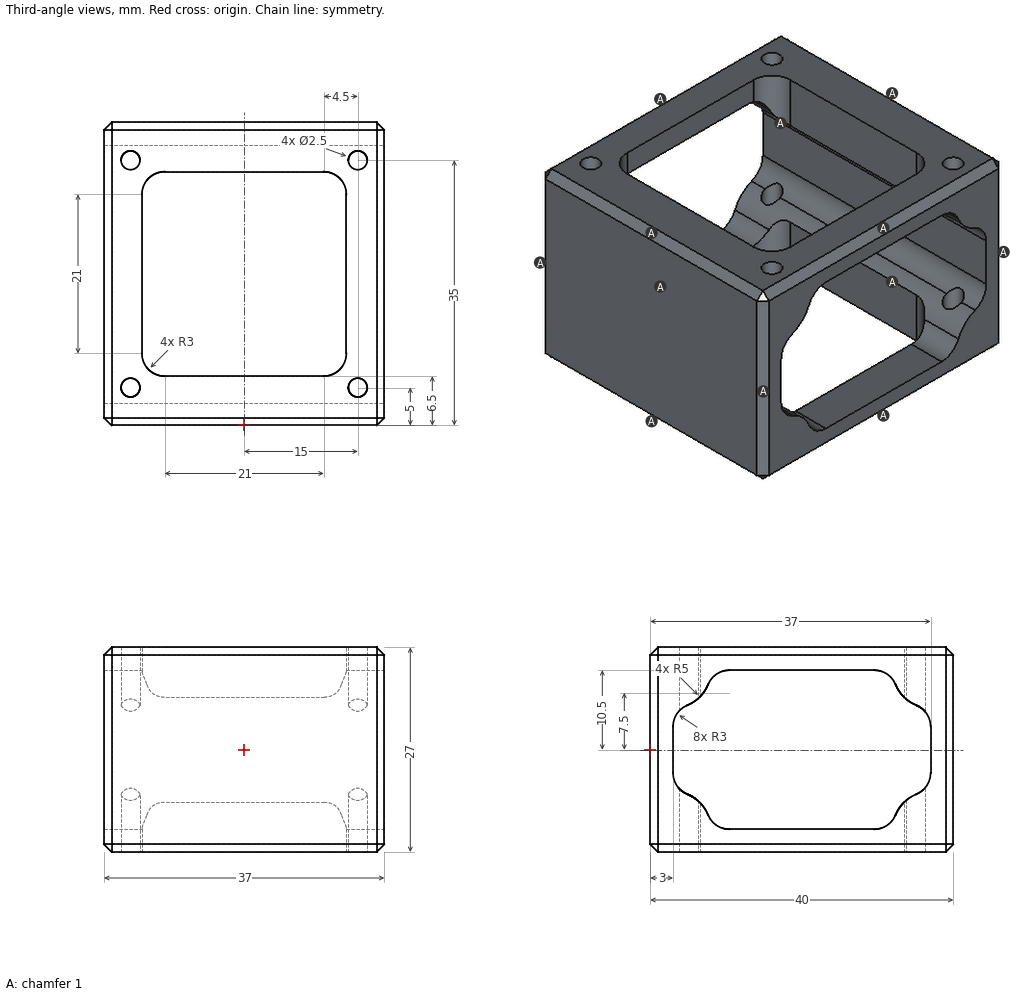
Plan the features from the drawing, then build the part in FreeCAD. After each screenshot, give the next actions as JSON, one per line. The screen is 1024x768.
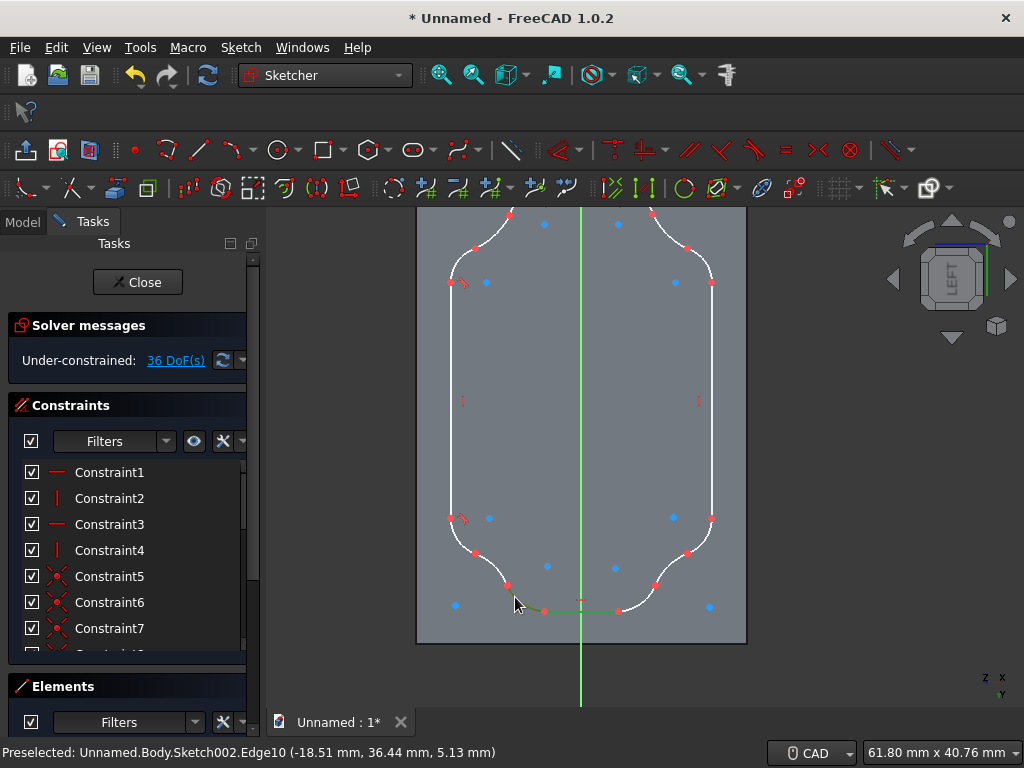
{"action": "left_click", "coordinate": [754, 150]}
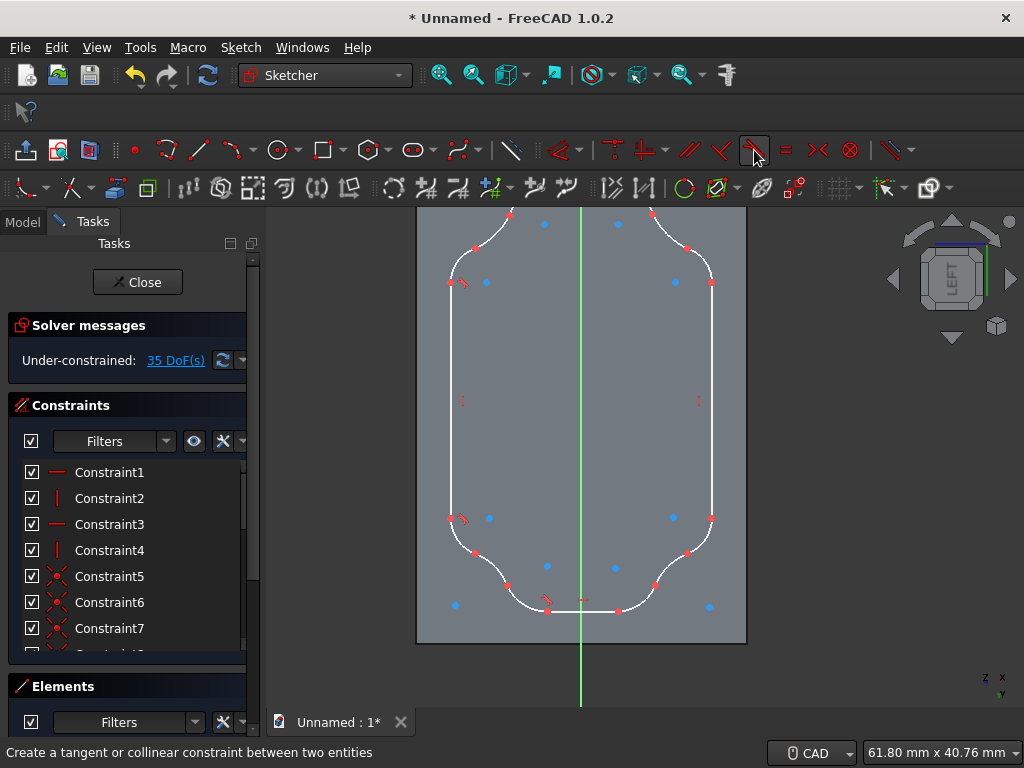
{"action": "left_click", "coordinate": [569, 612]}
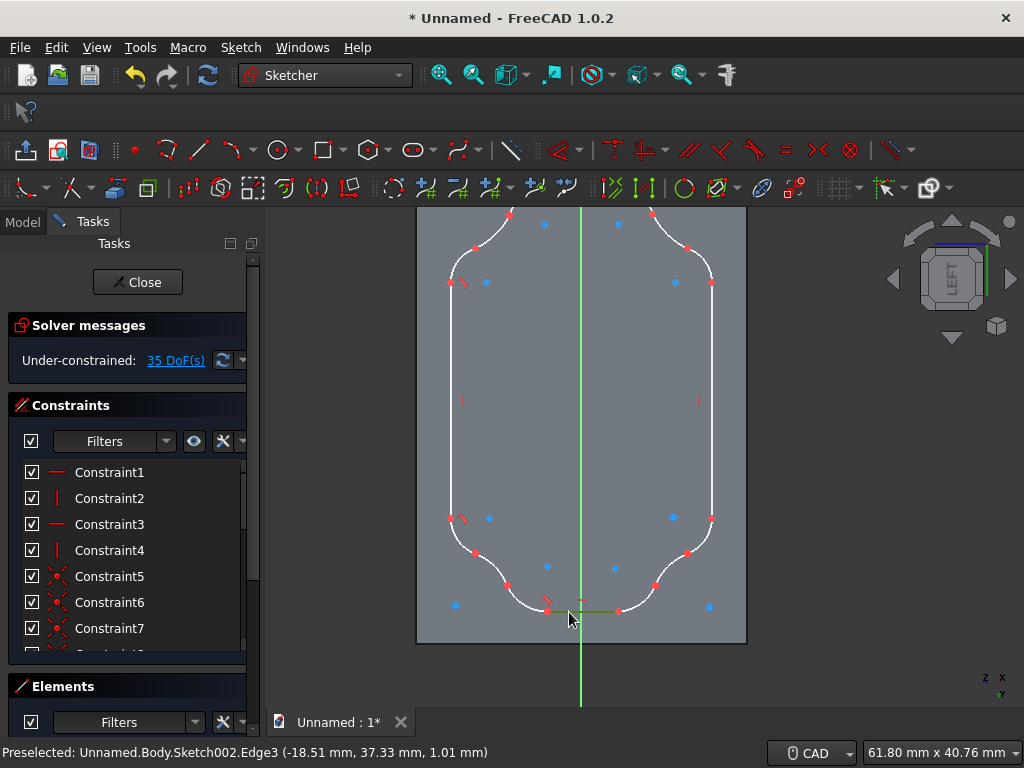
{"action": "left_click", "coordinate": [632, 608]}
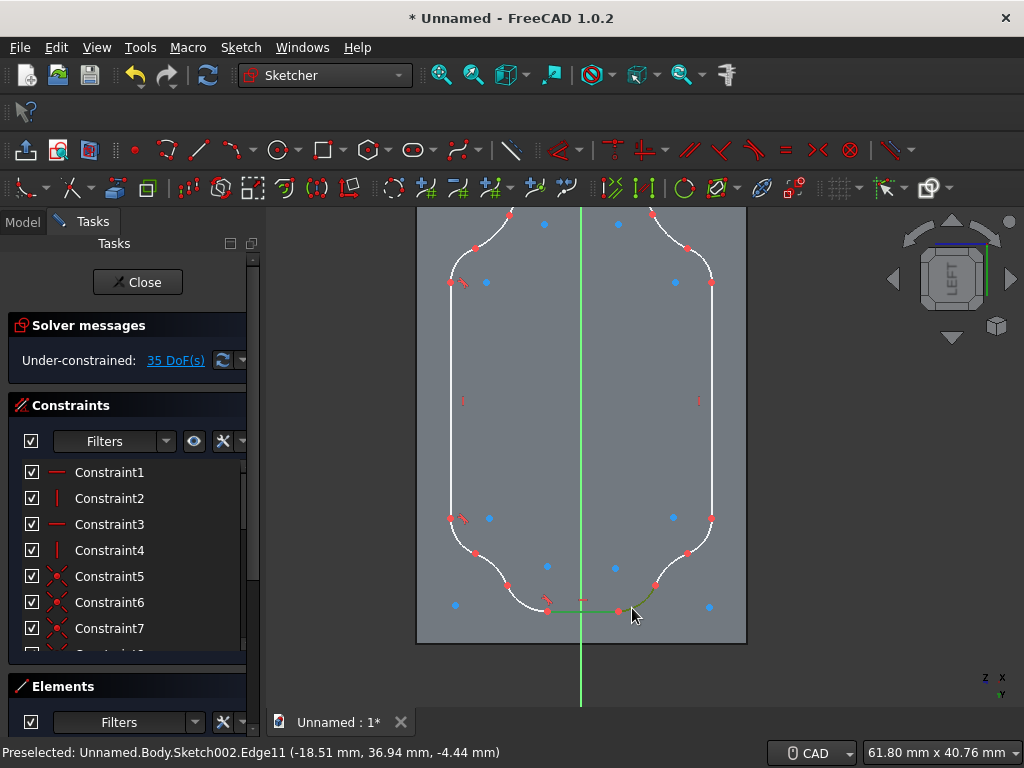
{"action": "left_click", "coordinate": [754, 150]}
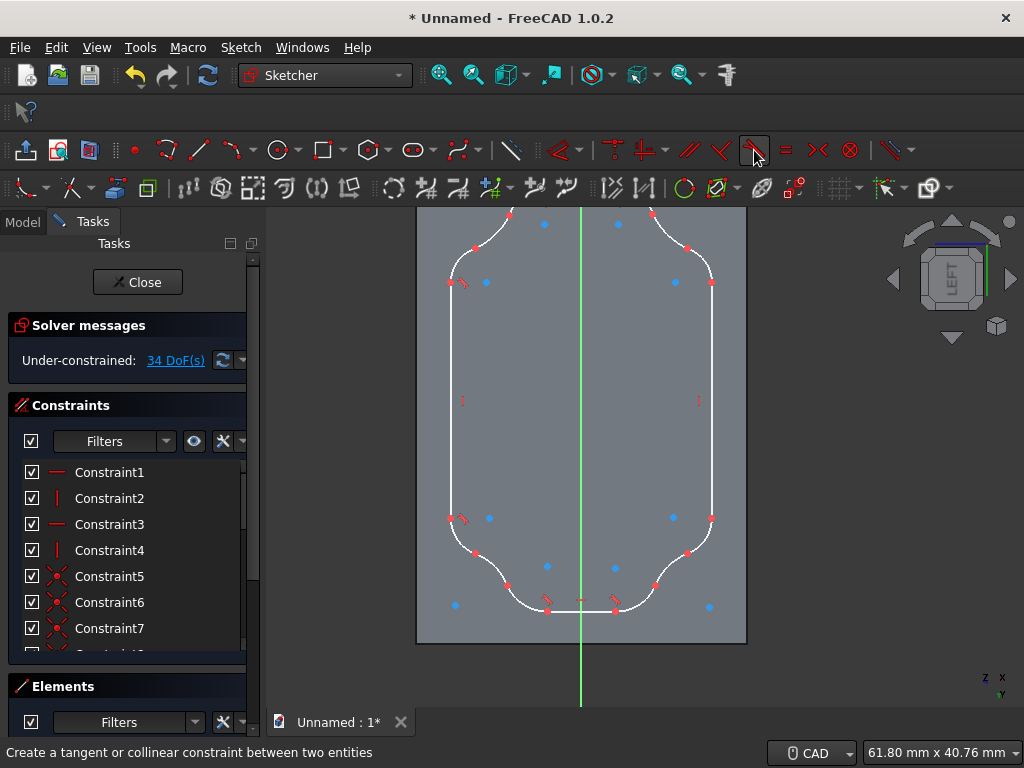
{"action": "left_click", "coordinate": [712, 448]}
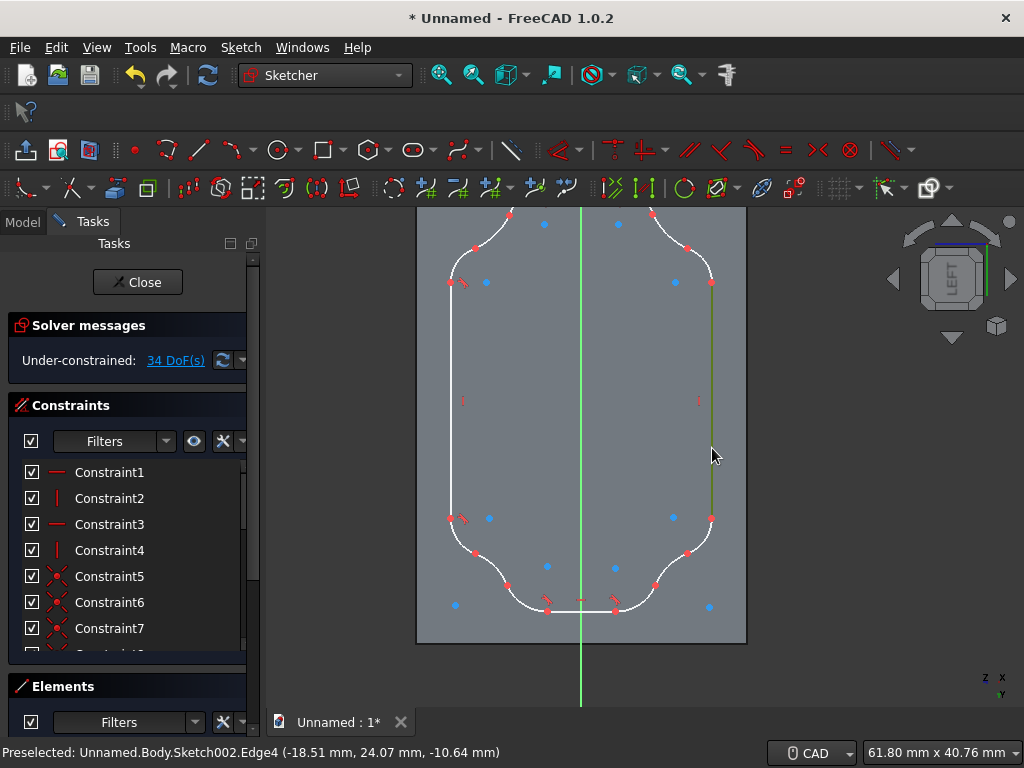
{"action": "left_click", "coordinate": [699, 547]}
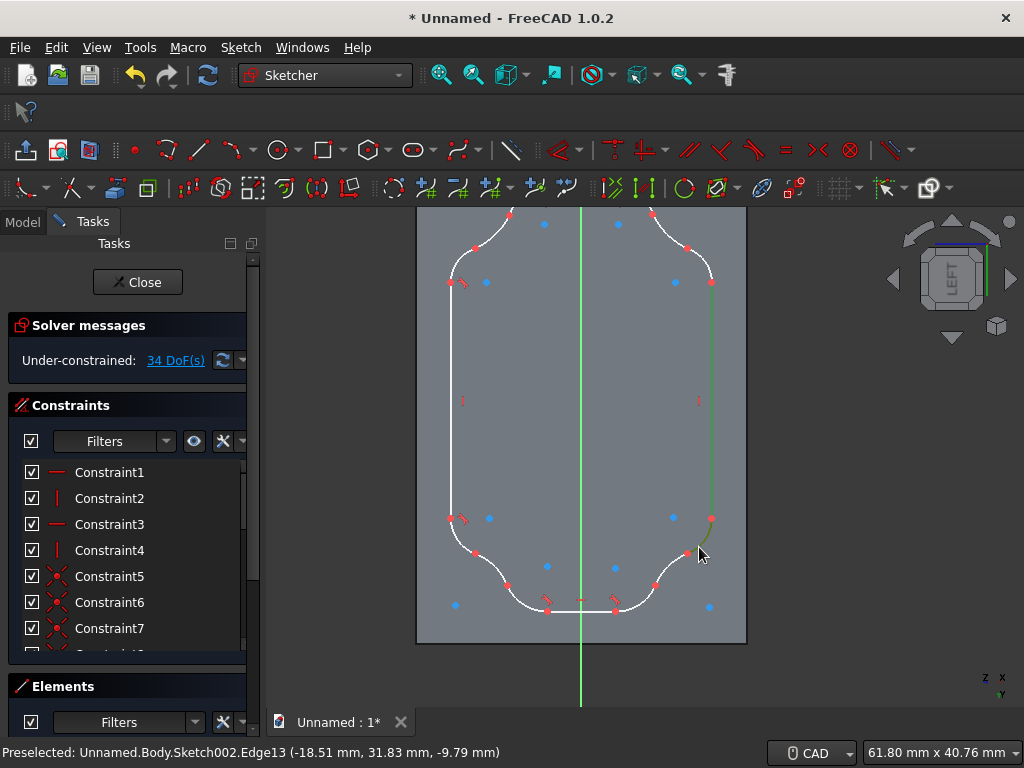
{"action": "left_click", "coordinate": [754, 150]}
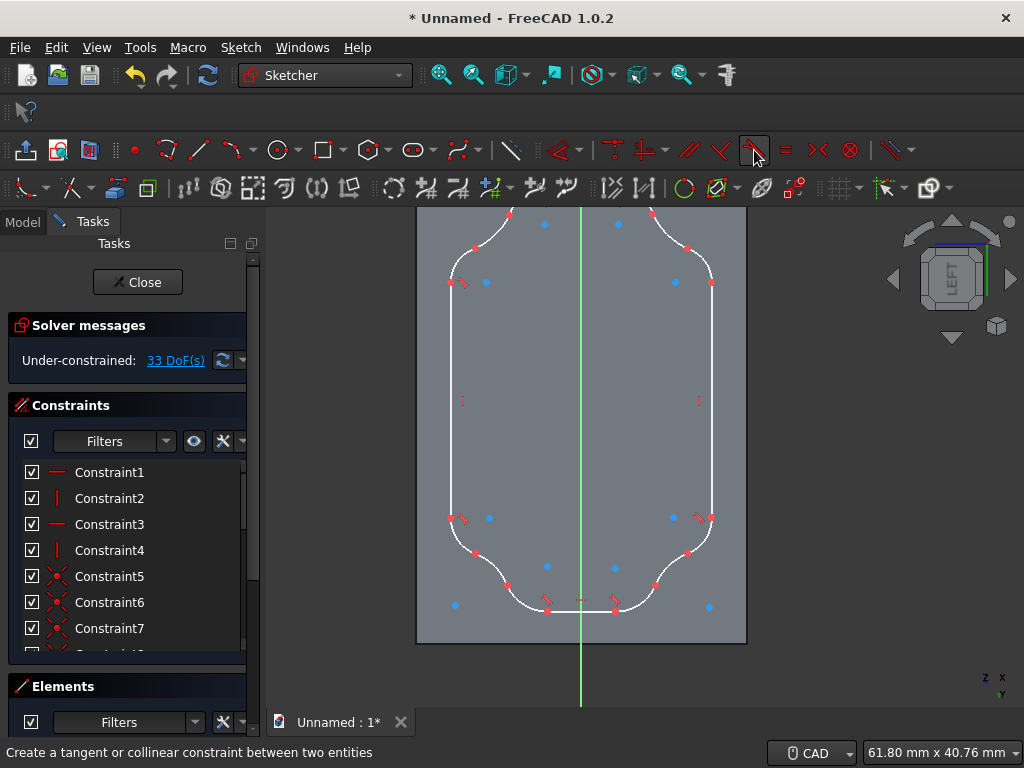
{"action": "left_click", "coordinate": [712, 447]}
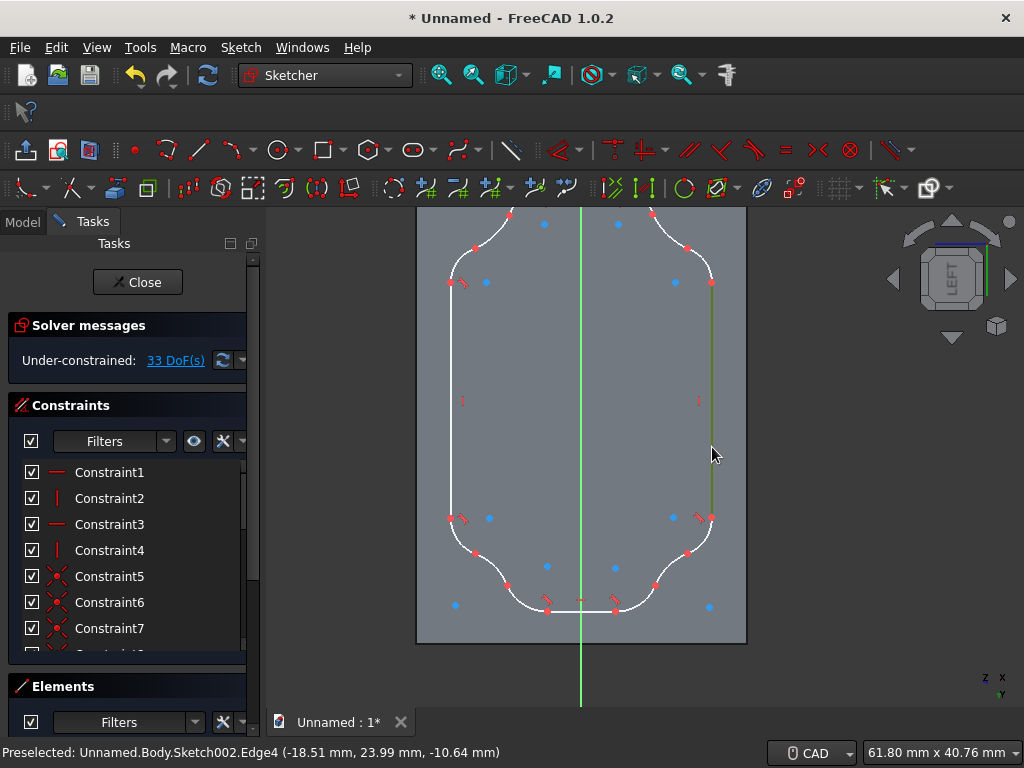
{"action": "left_click", "coordinate": [709, 269]}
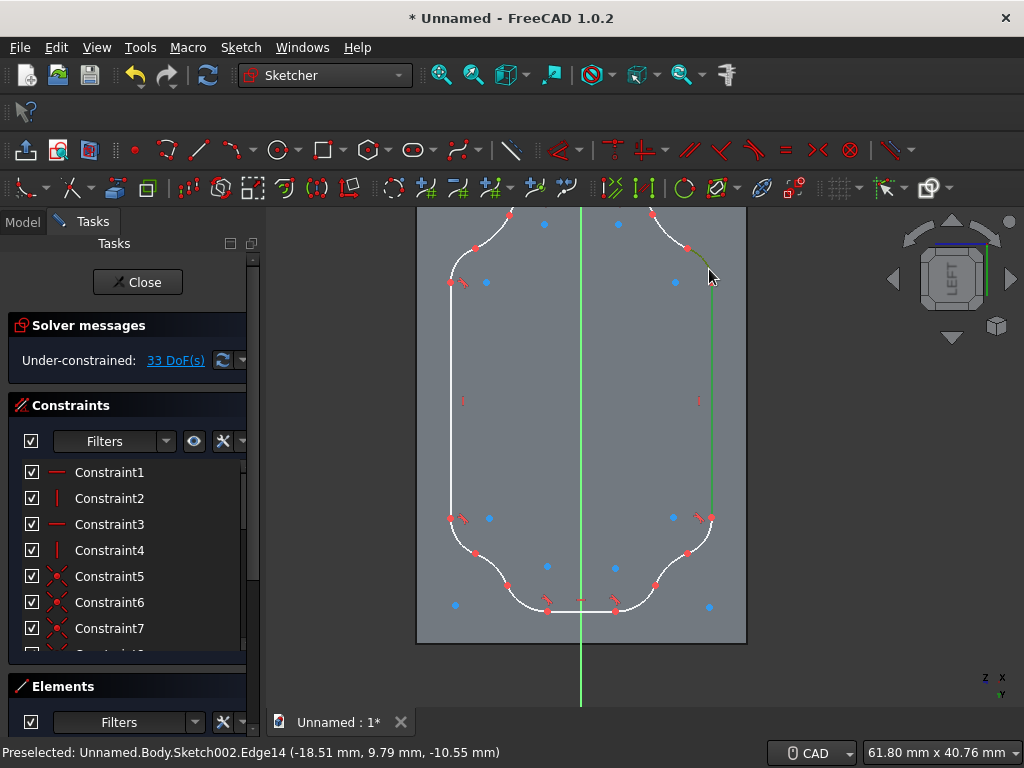
{"action": "key", "text": "t"}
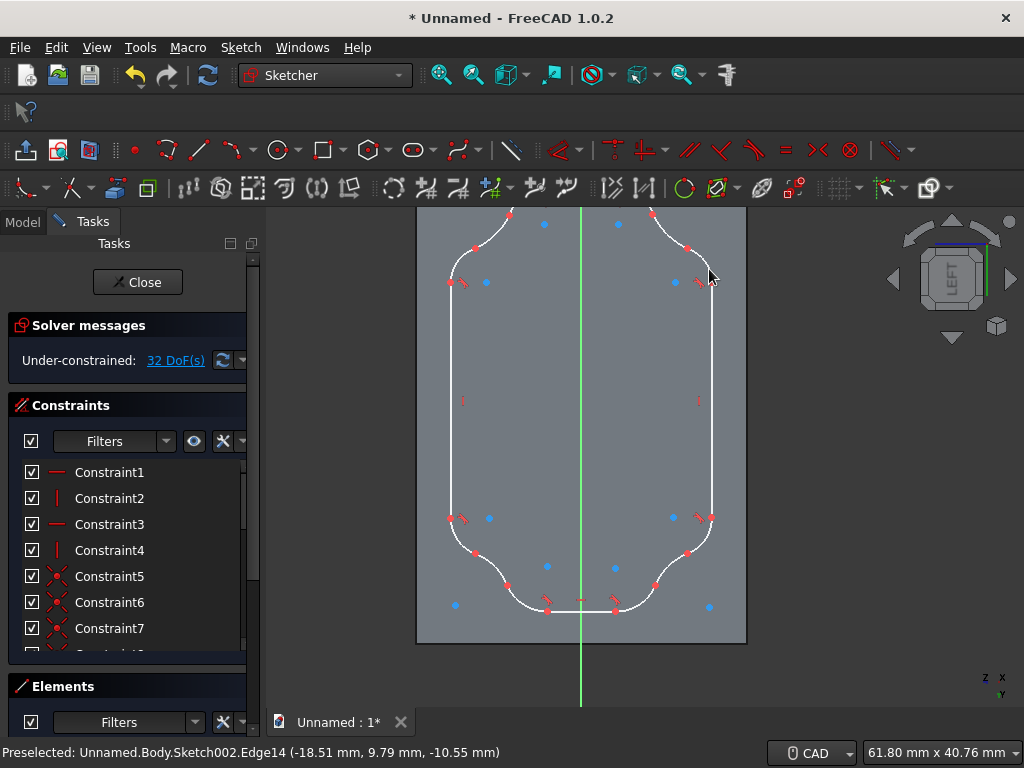
{"action": "scroll", "coordinate": [567, 612], "scroll_direction": "down", "scroll_amount": 2}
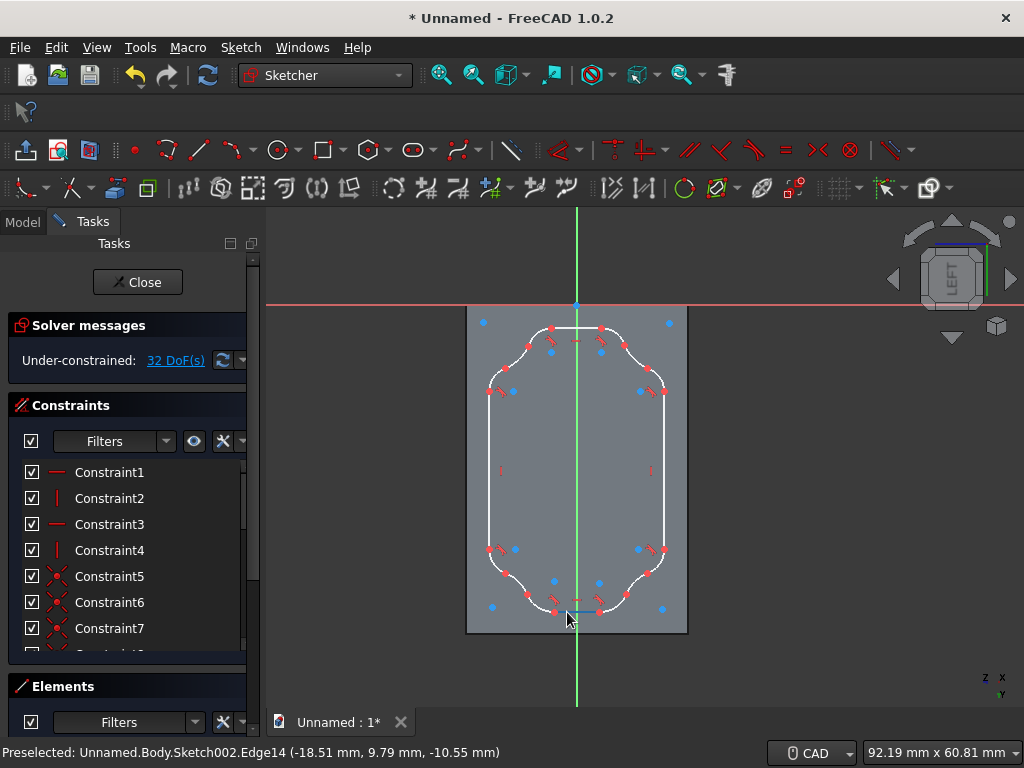
{"action": "scroll", "coordinate": [543, 330], "scroll_direction": "up", "scroll_amount": 2}